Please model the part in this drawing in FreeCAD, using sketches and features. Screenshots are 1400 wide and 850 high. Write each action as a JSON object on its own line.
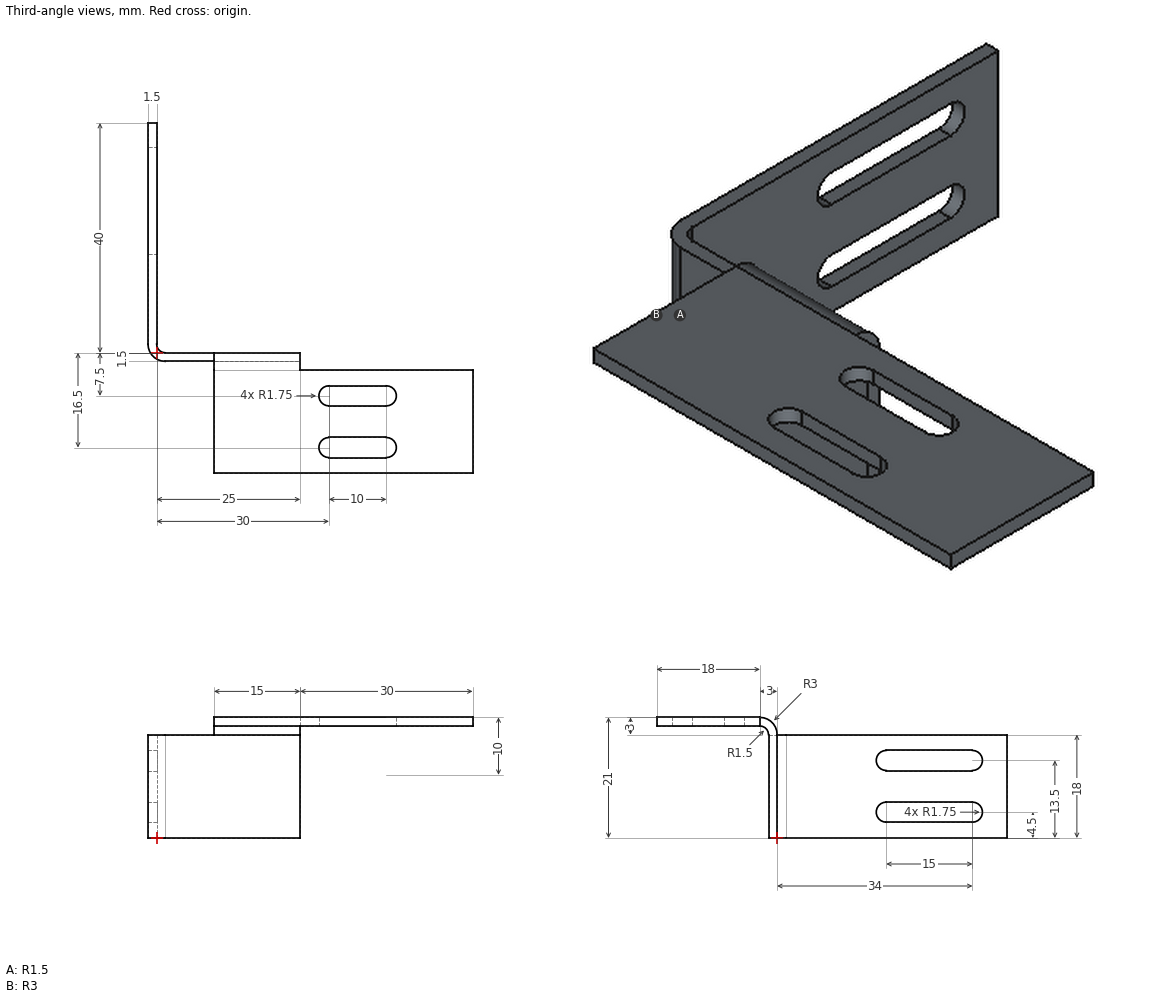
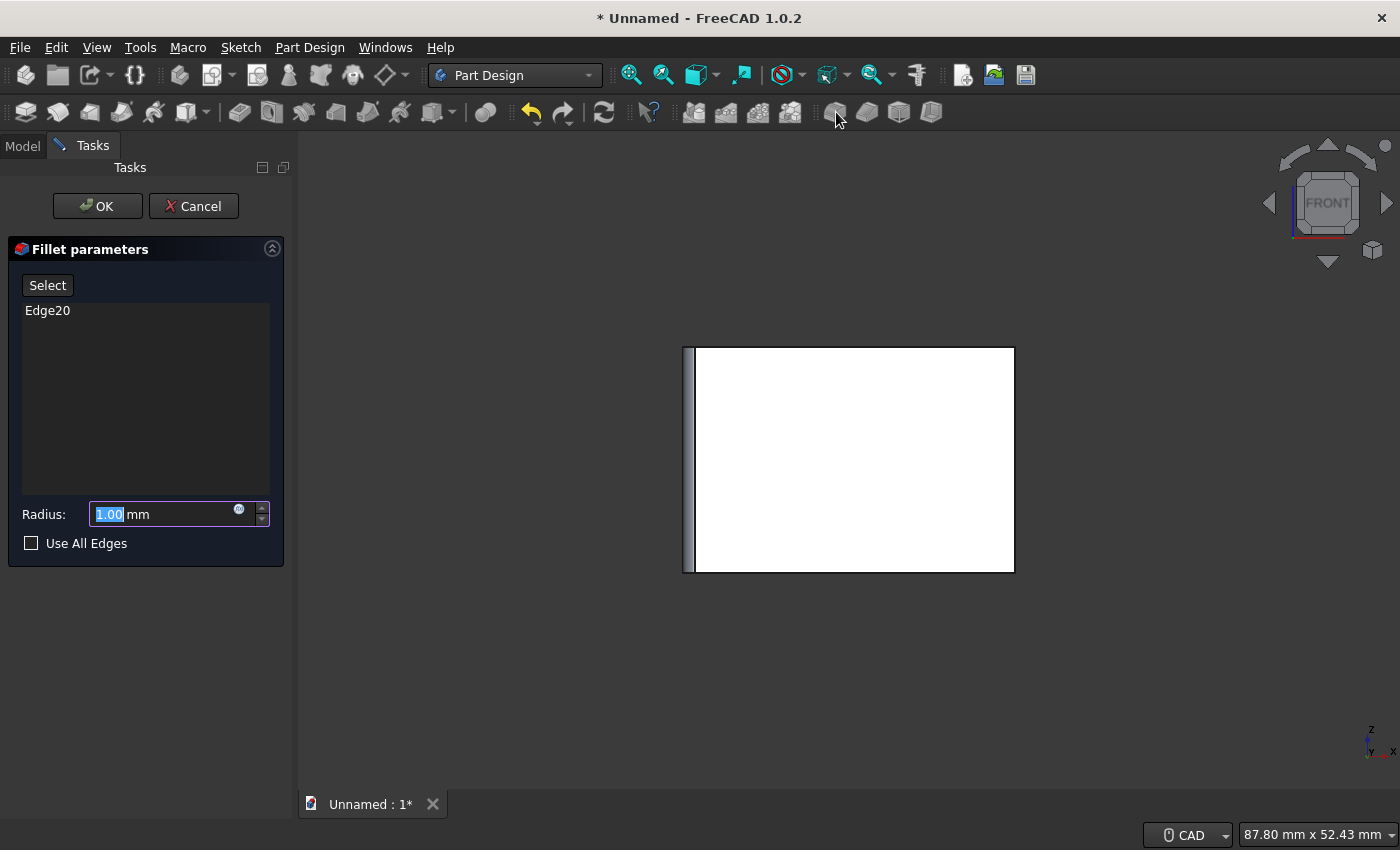
{"action": "type", "text": "3"}
{"action": "key", "text": "Tab"}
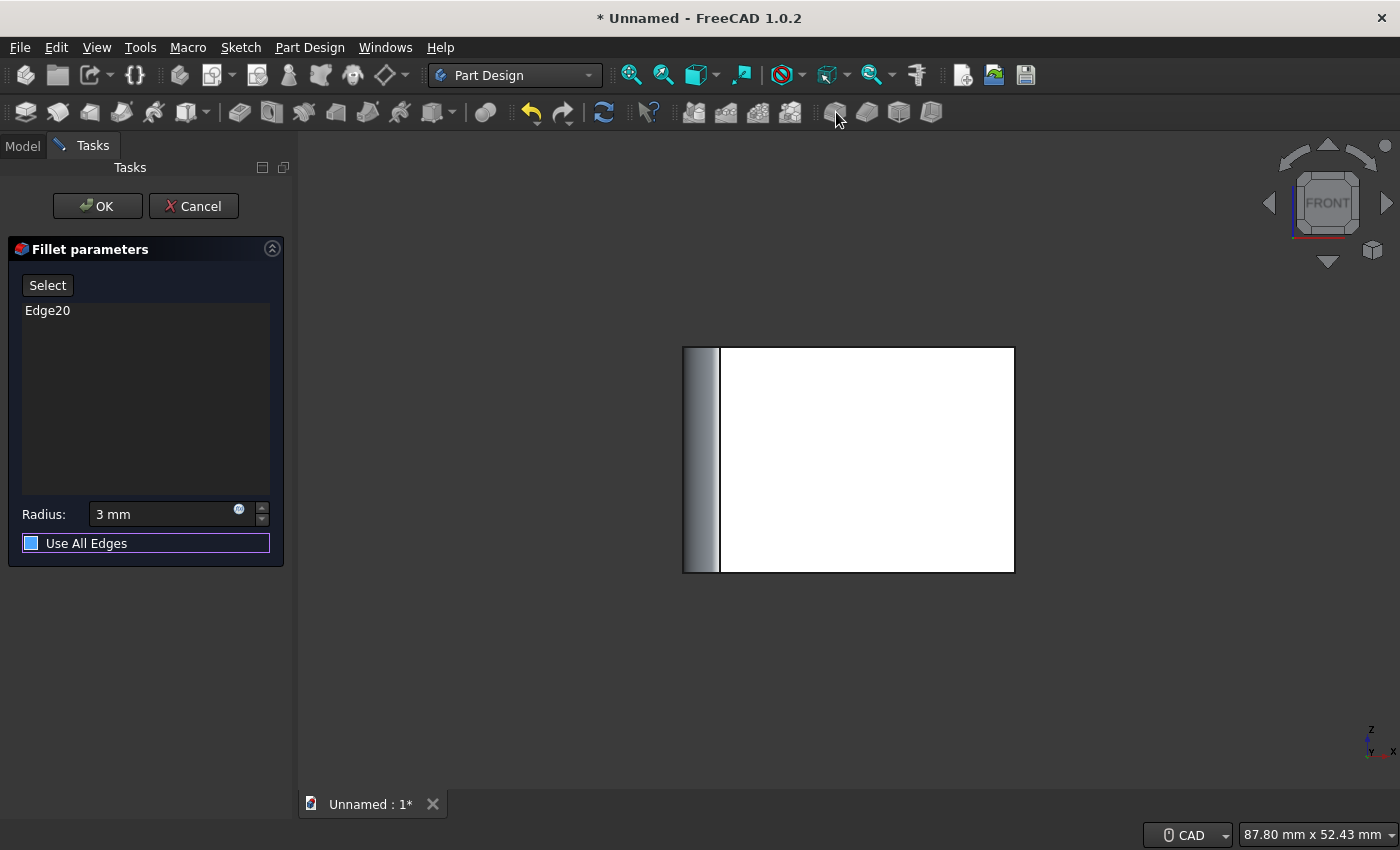
{"action": "left_click", "coordinate": [98, 206]}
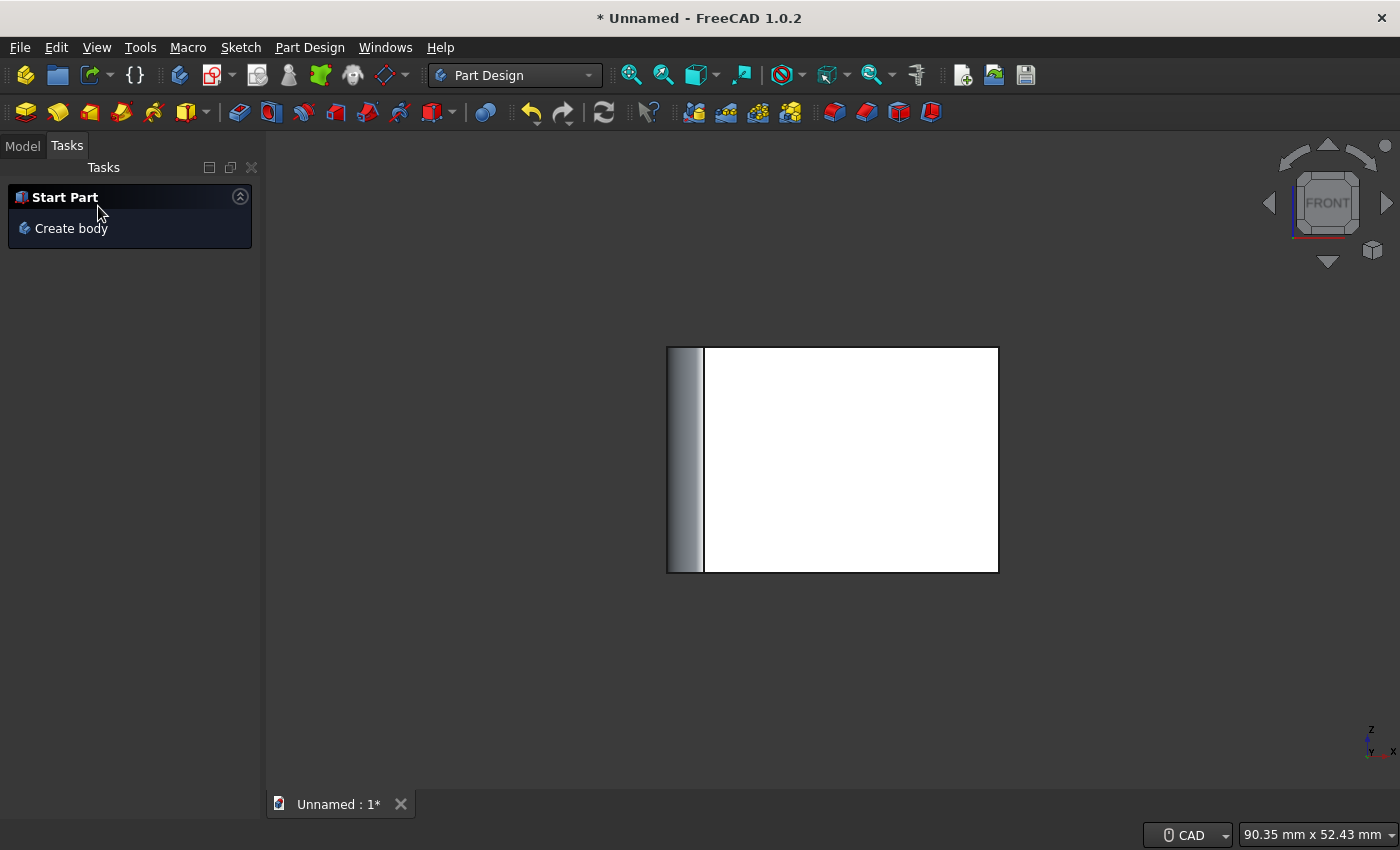
{"action": "key", "text": "v f"}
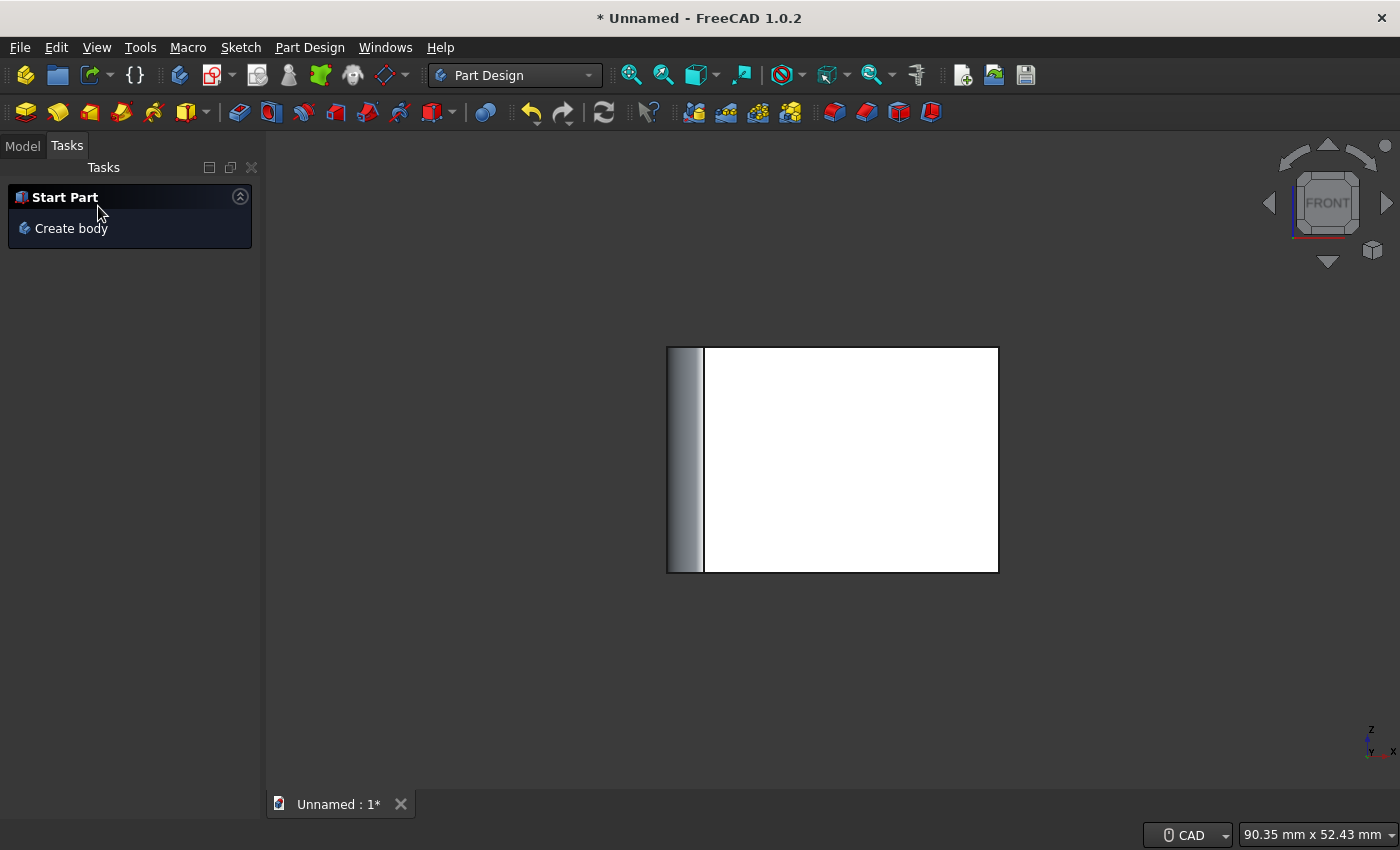
{"action": "key", "text": "0"}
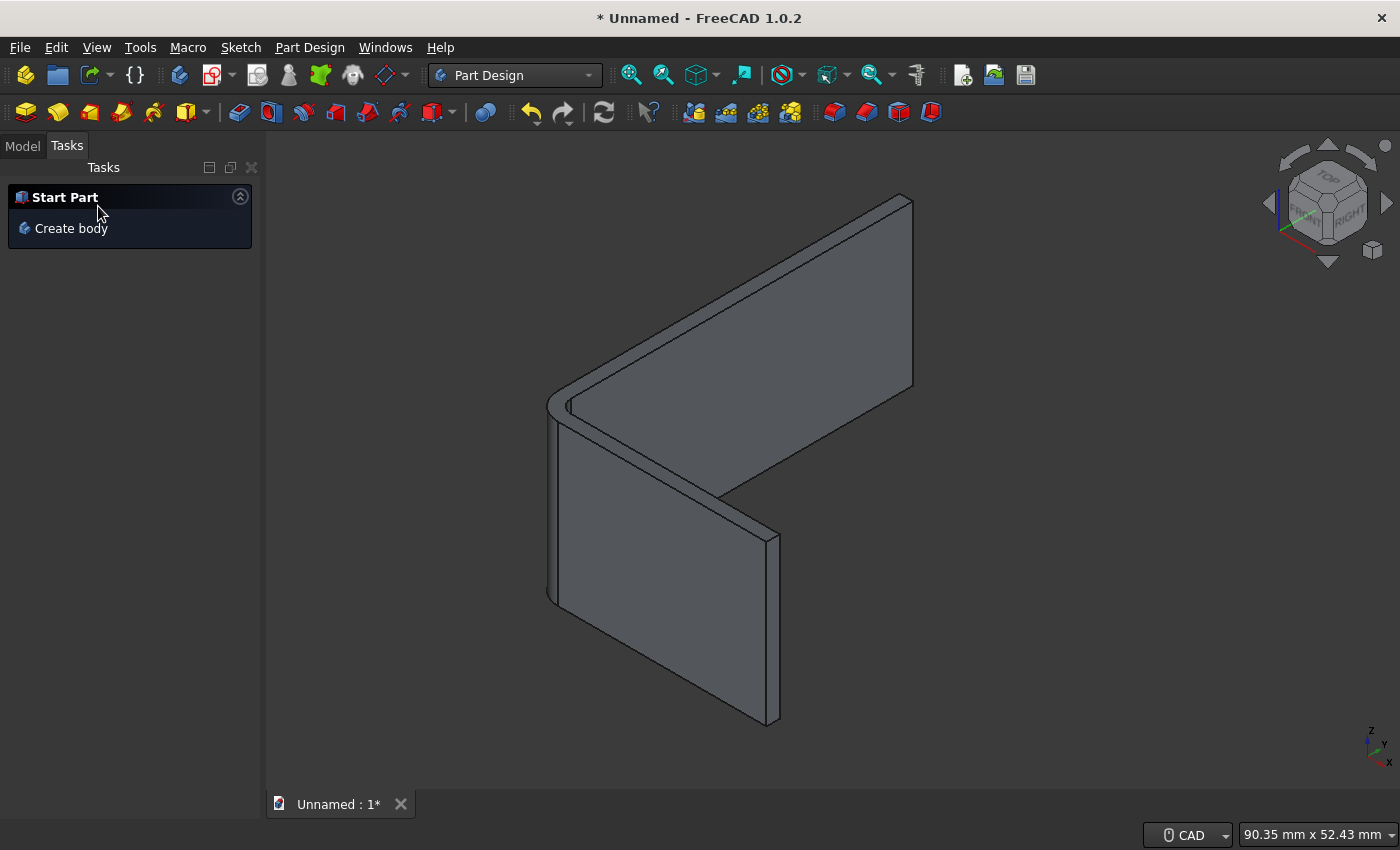
{"action": "left_click", "coordinate": [775, 549]}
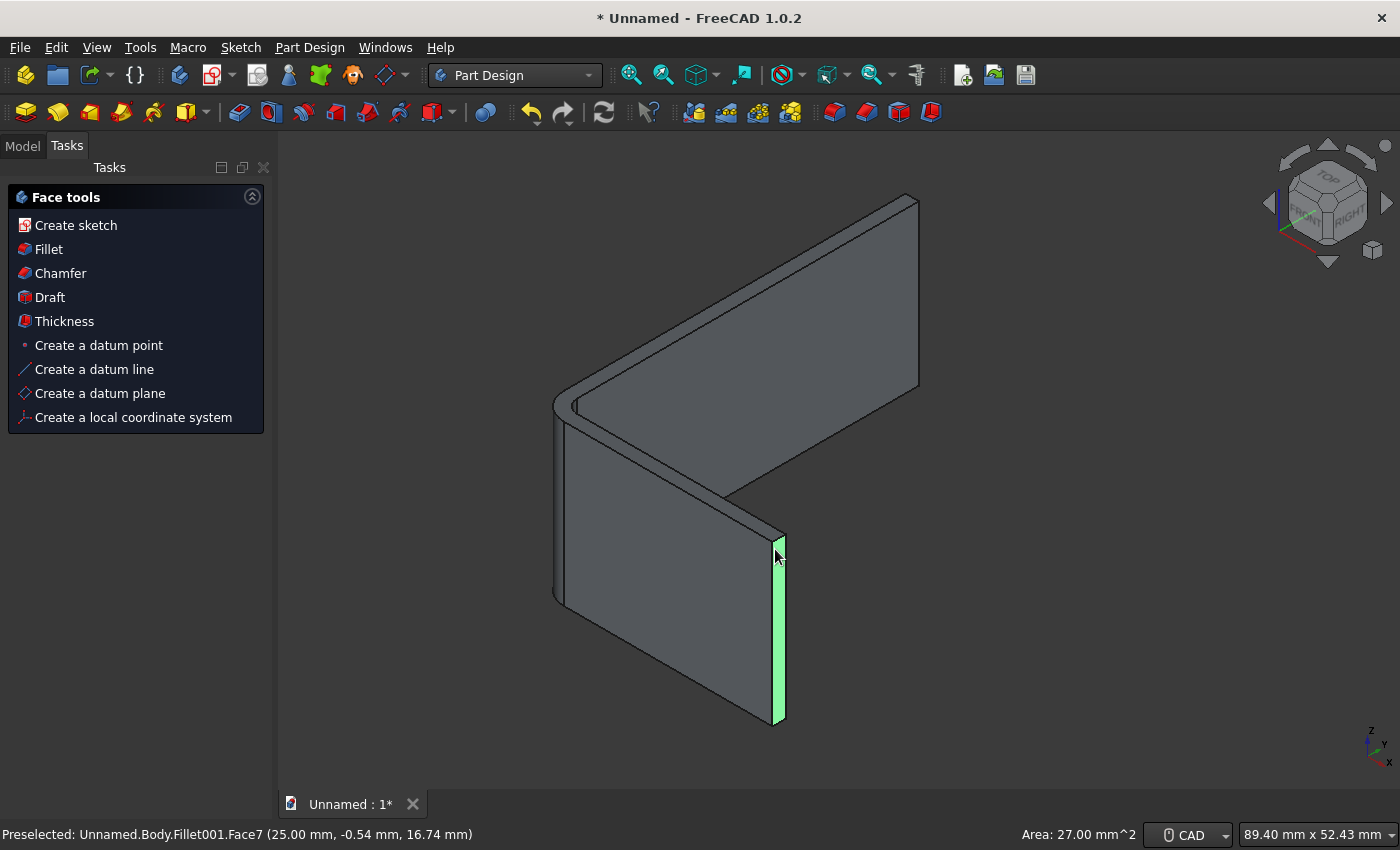
{"action": "left_click", "coordinate": [212, 76]}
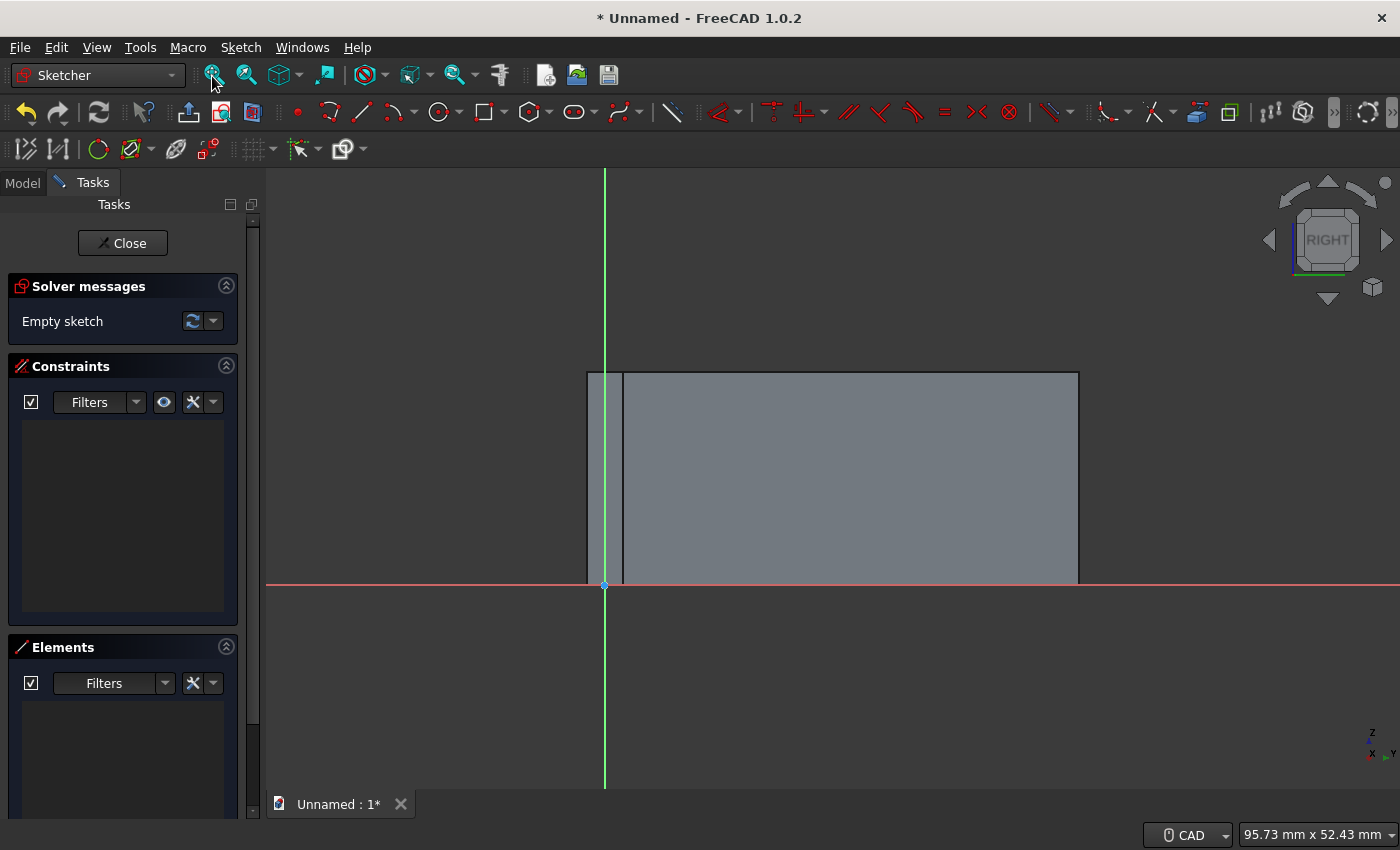
{"action": "scroll", "coordinate": [294, 425], "scroll_direction": "up", "scroll_amount": 2}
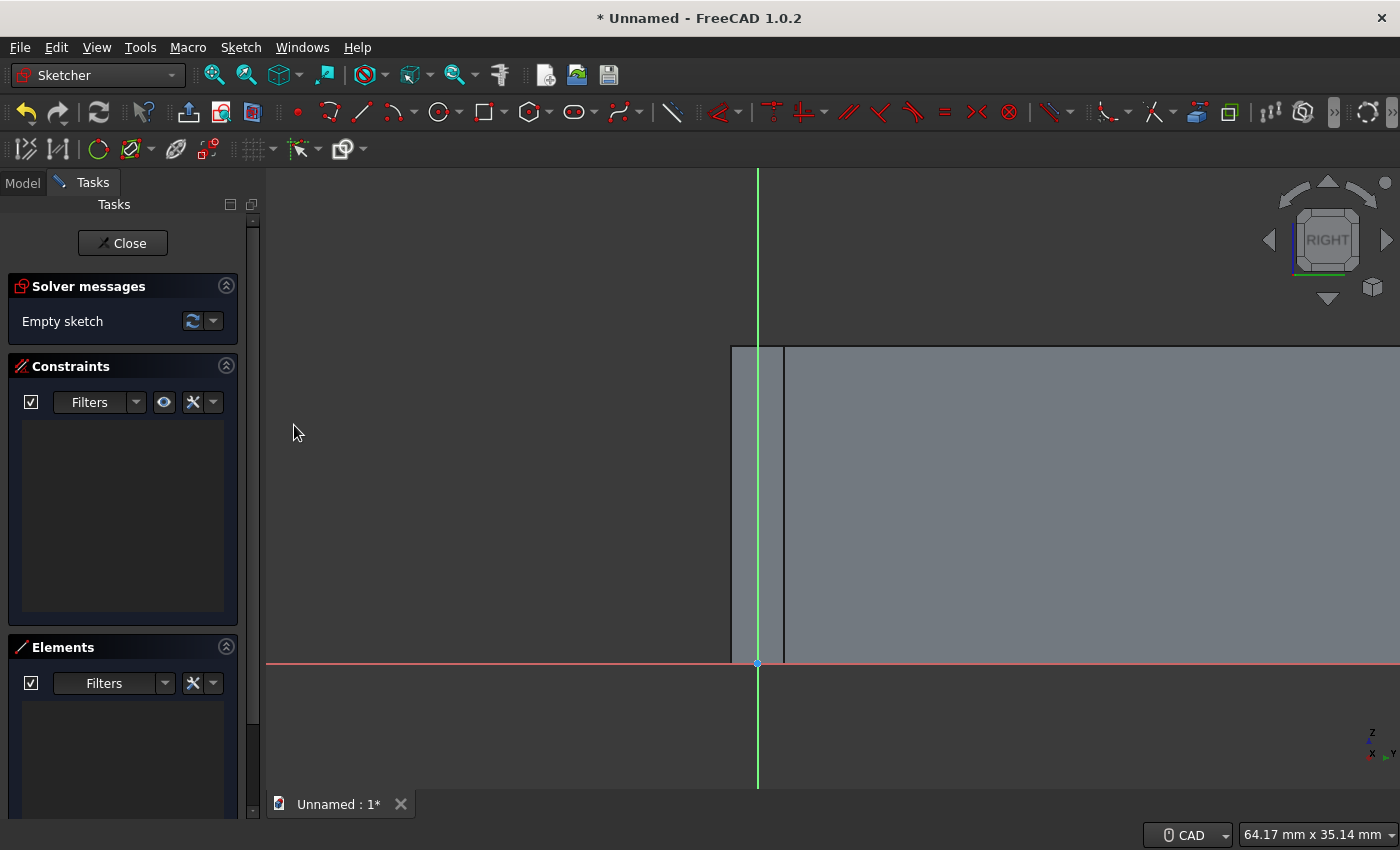
{"action": "key", "text": "g m"}